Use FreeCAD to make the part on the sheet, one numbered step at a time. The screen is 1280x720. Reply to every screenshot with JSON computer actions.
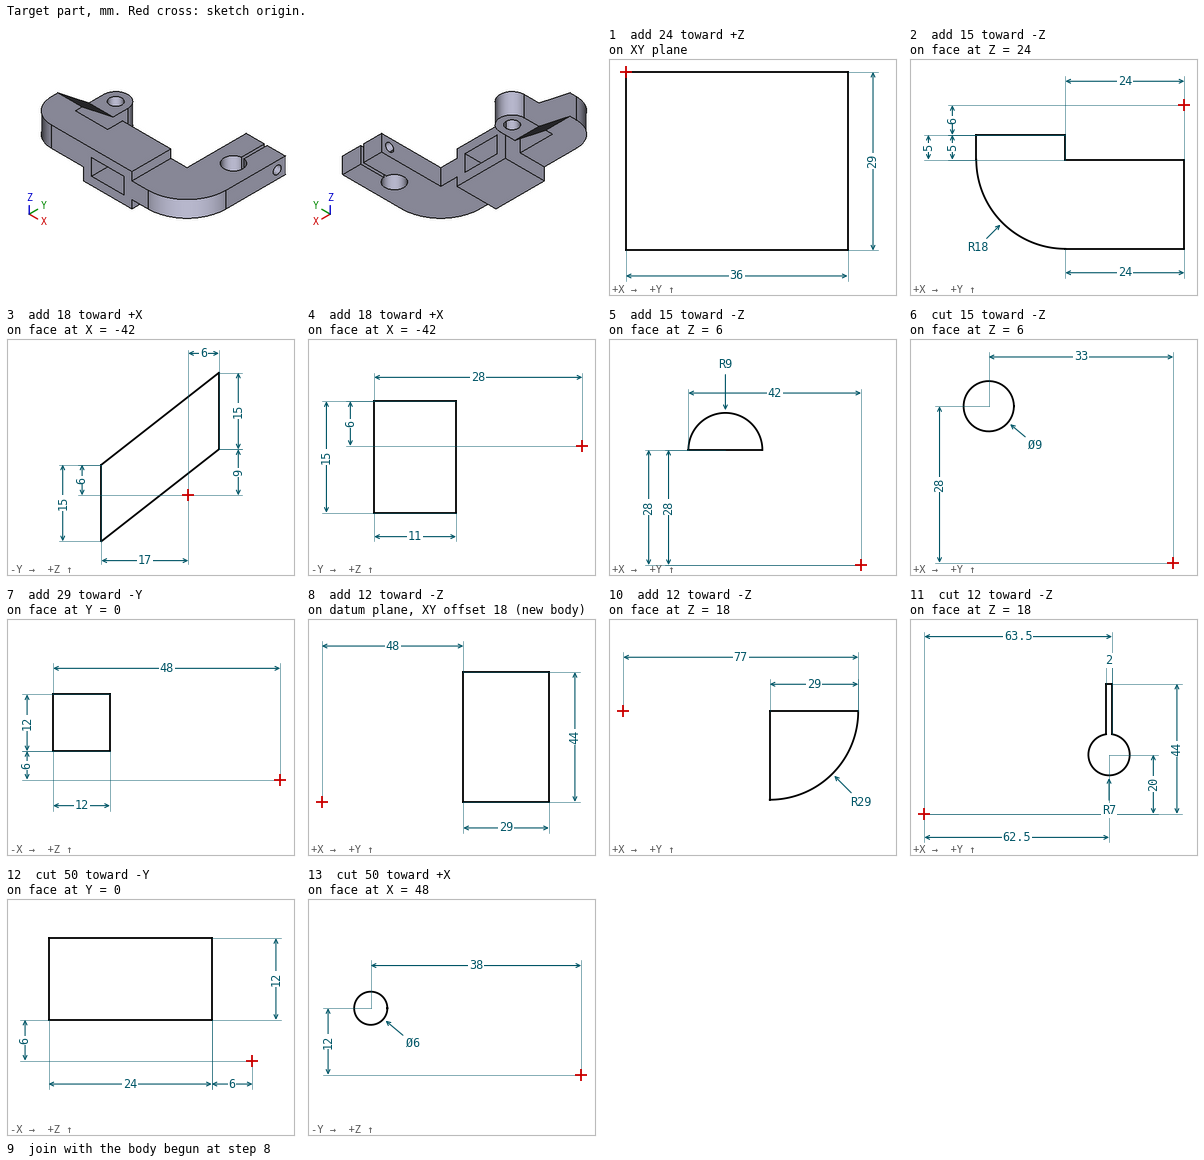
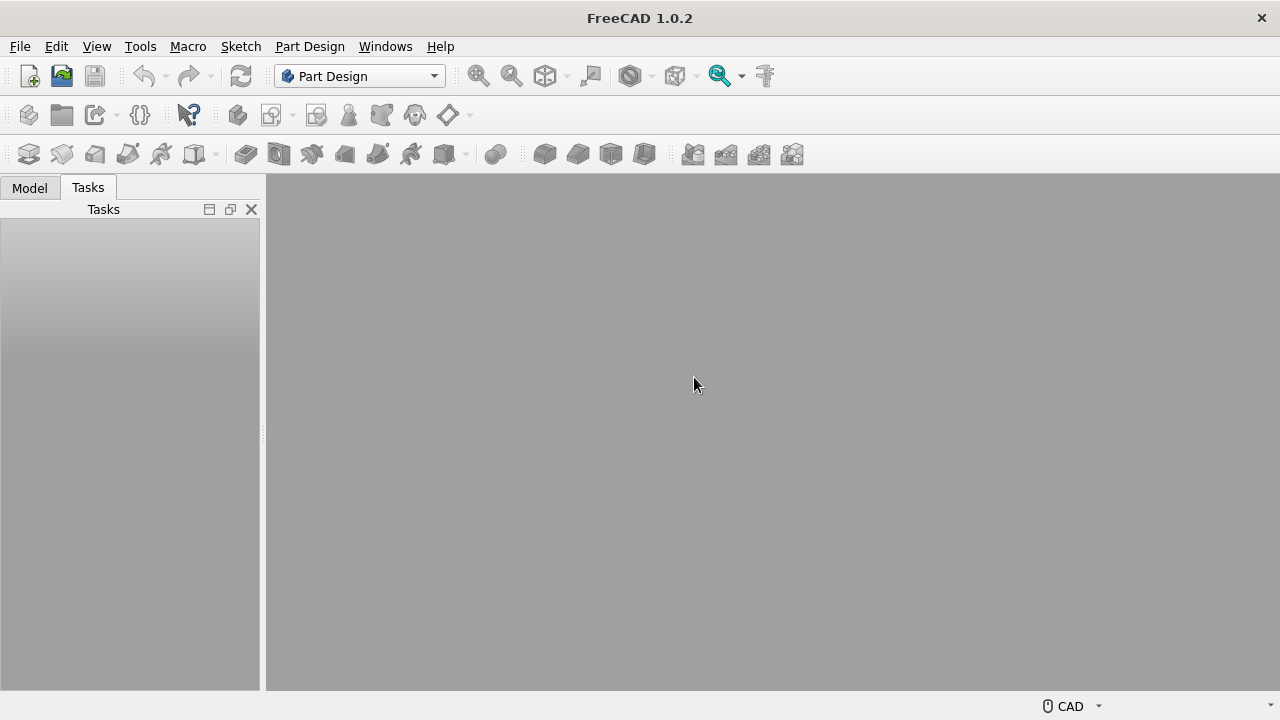
{"action": "key", "text": "ctrl+n"}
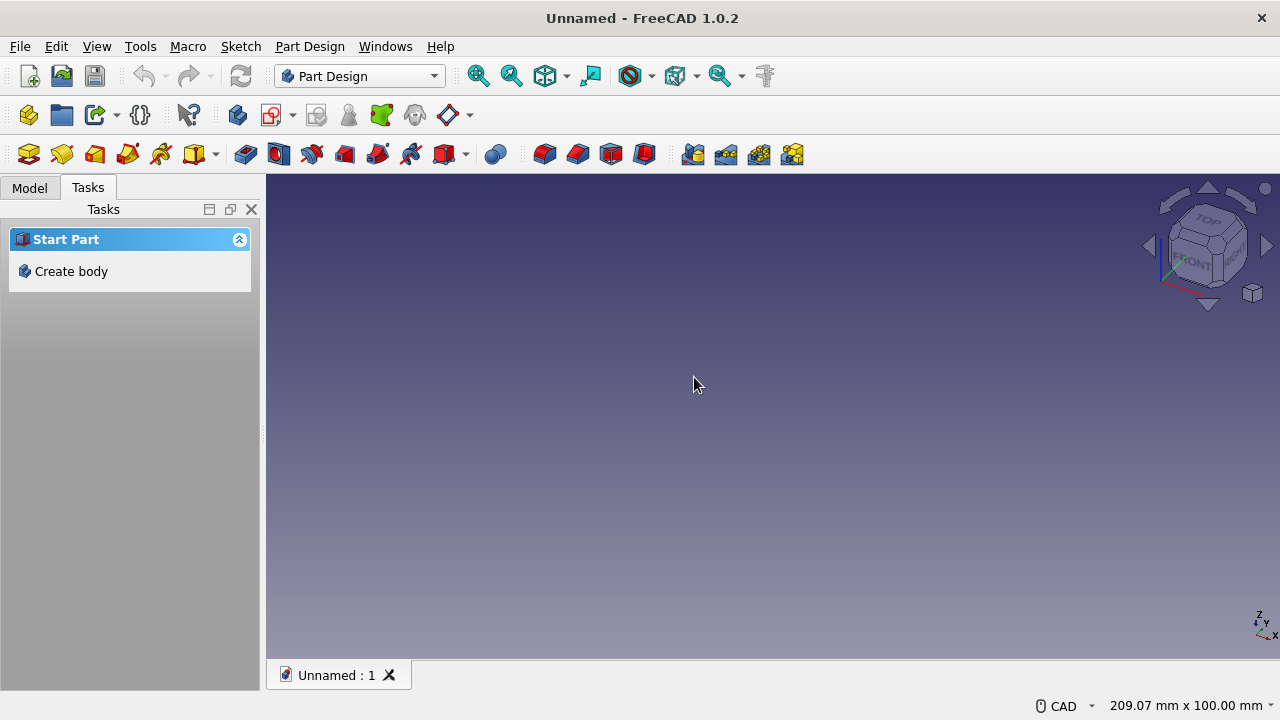
{"action": "left_click", "coordinate": [270, 116]}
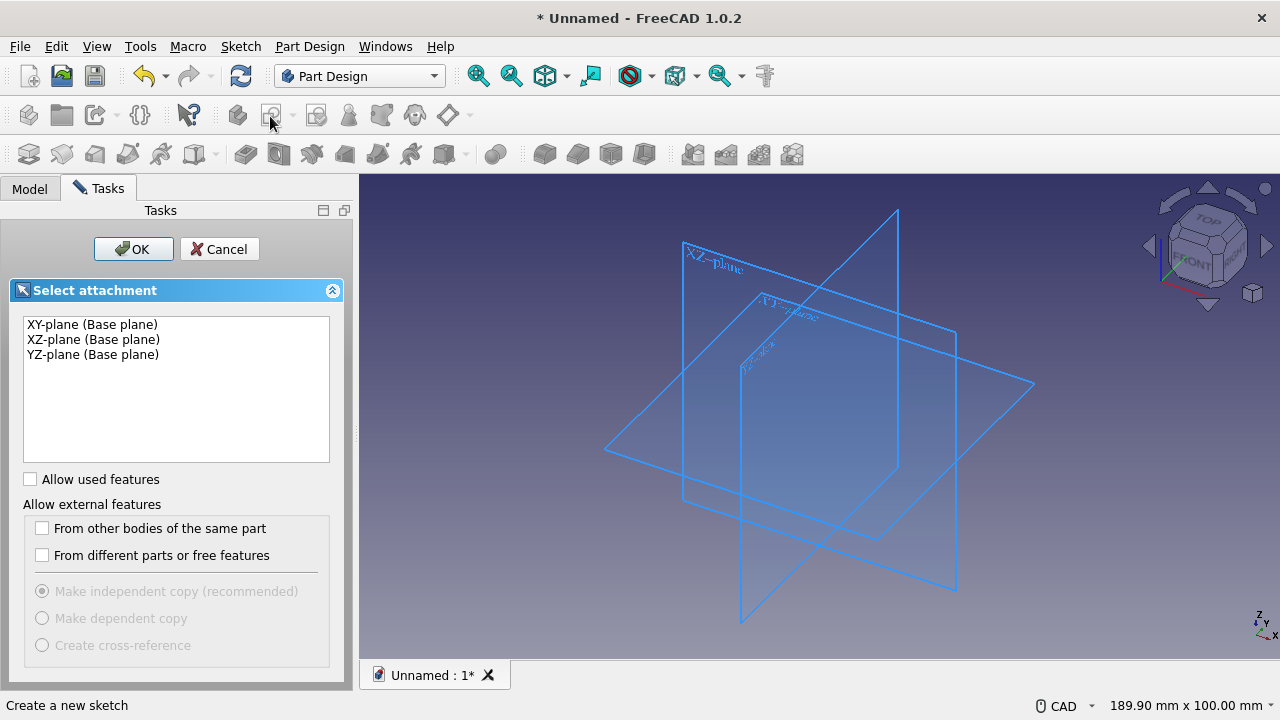
{"action": "left_click", "coordinate": [84, 324]}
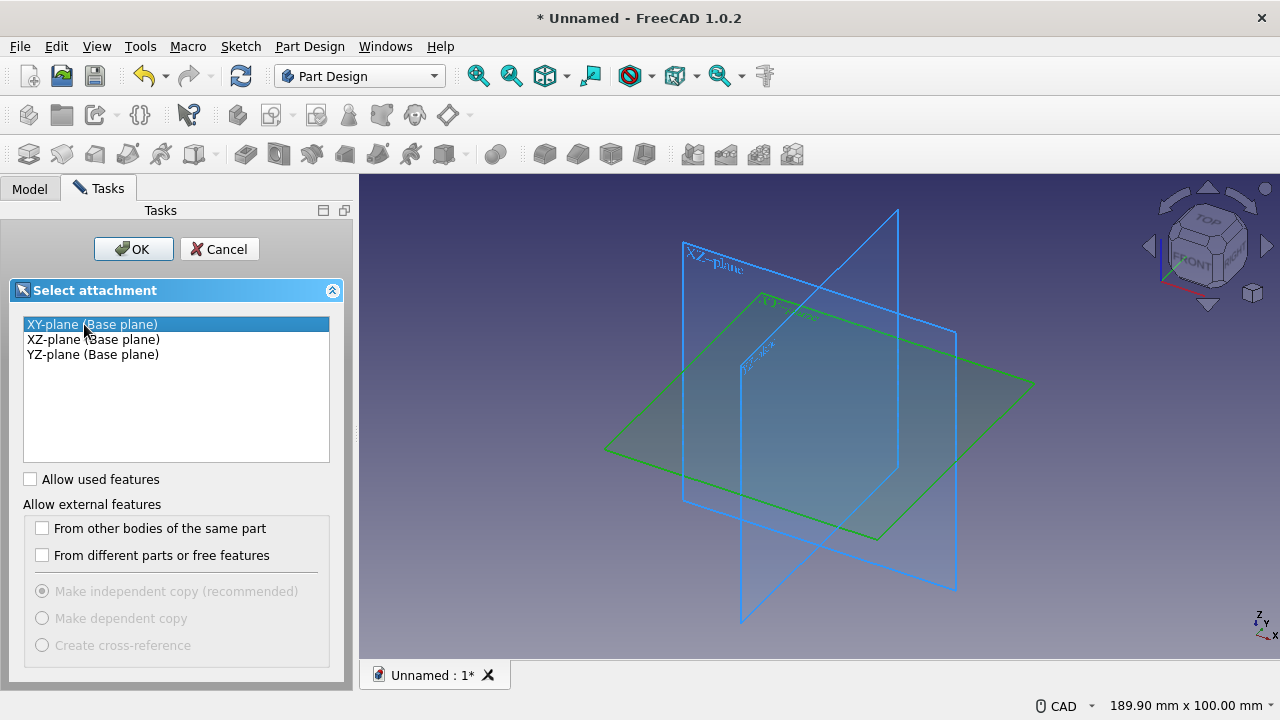
{"action": "left_click", "coordinate": [134, 249]}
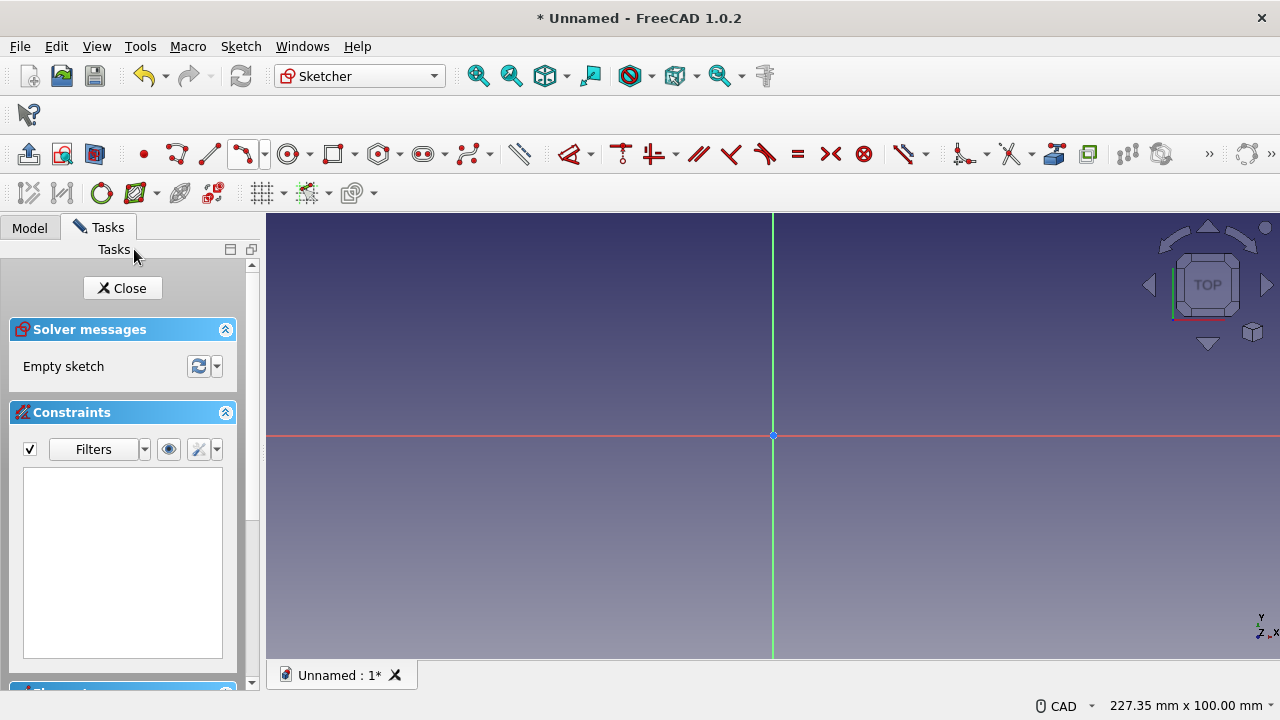
{"action": "scroll", "coordinate": [975, 553], "scroll_direction": "up", "scroll_amount": 4}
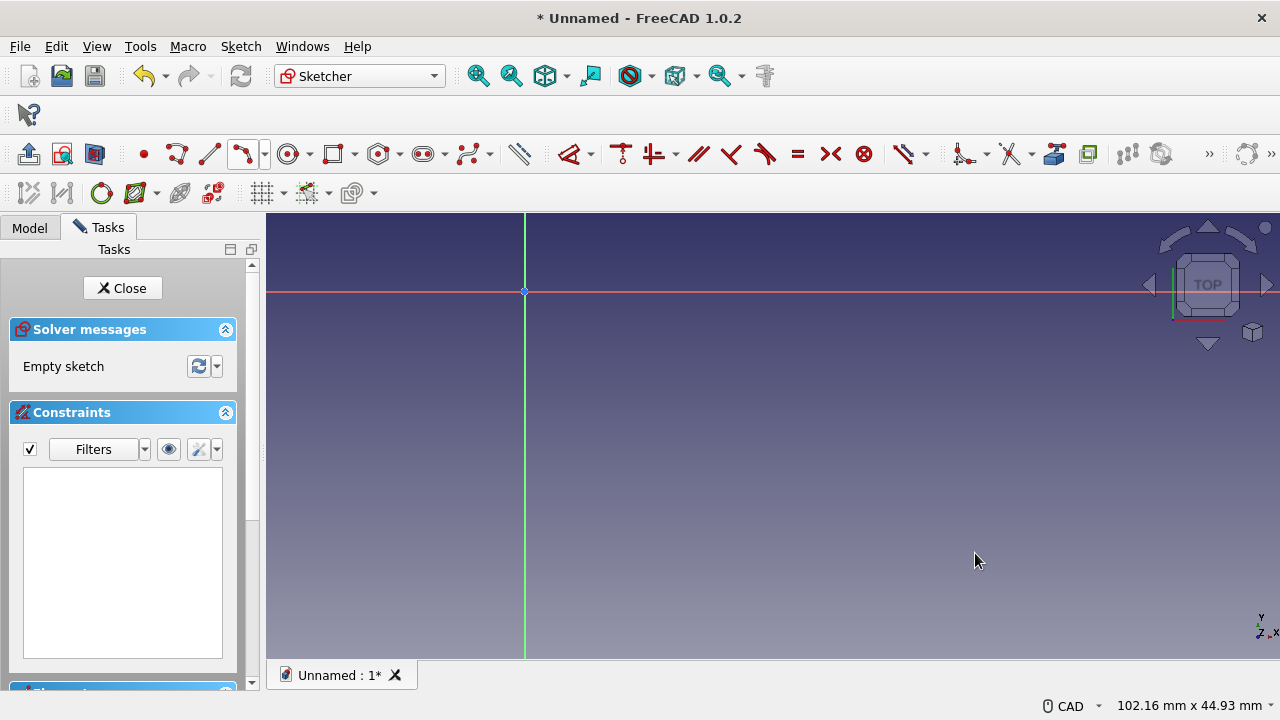
{"action": "left_click", "coordinate": [332, 154]}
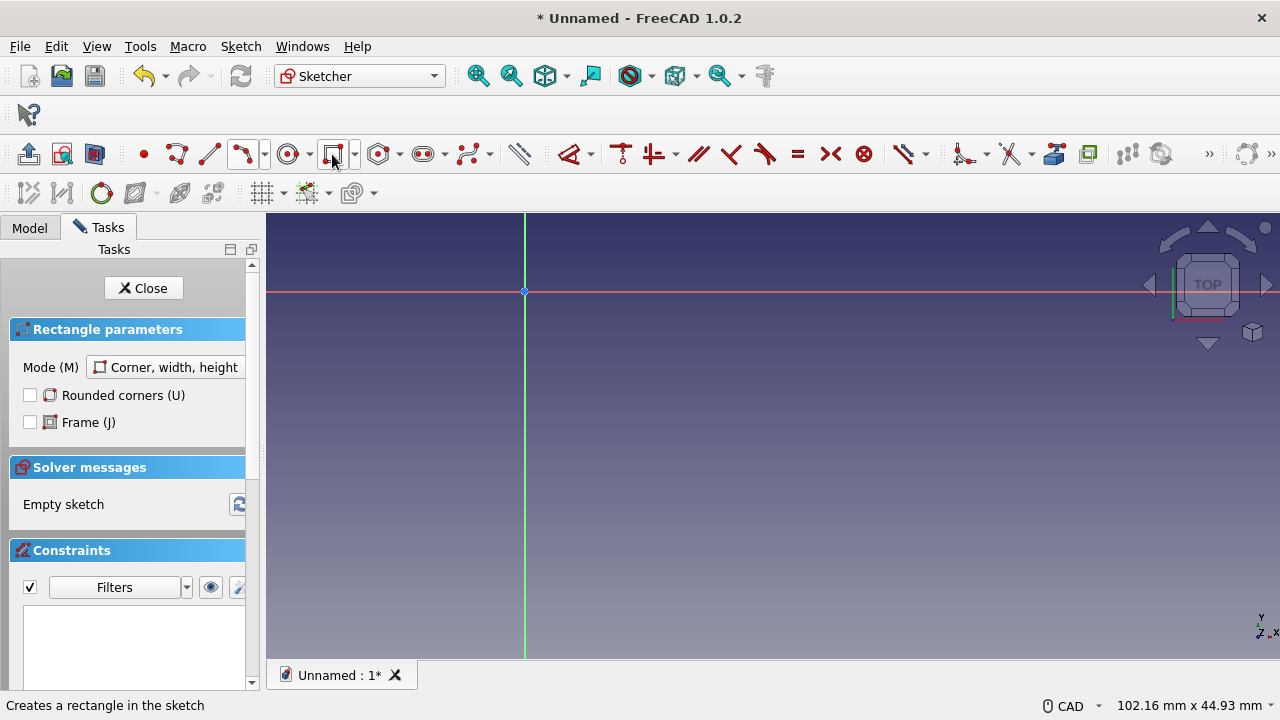
{"action": "left_click", "coordinate": [525, 292]}
{"action": "mouse_move", "coordinate": [882, 580]}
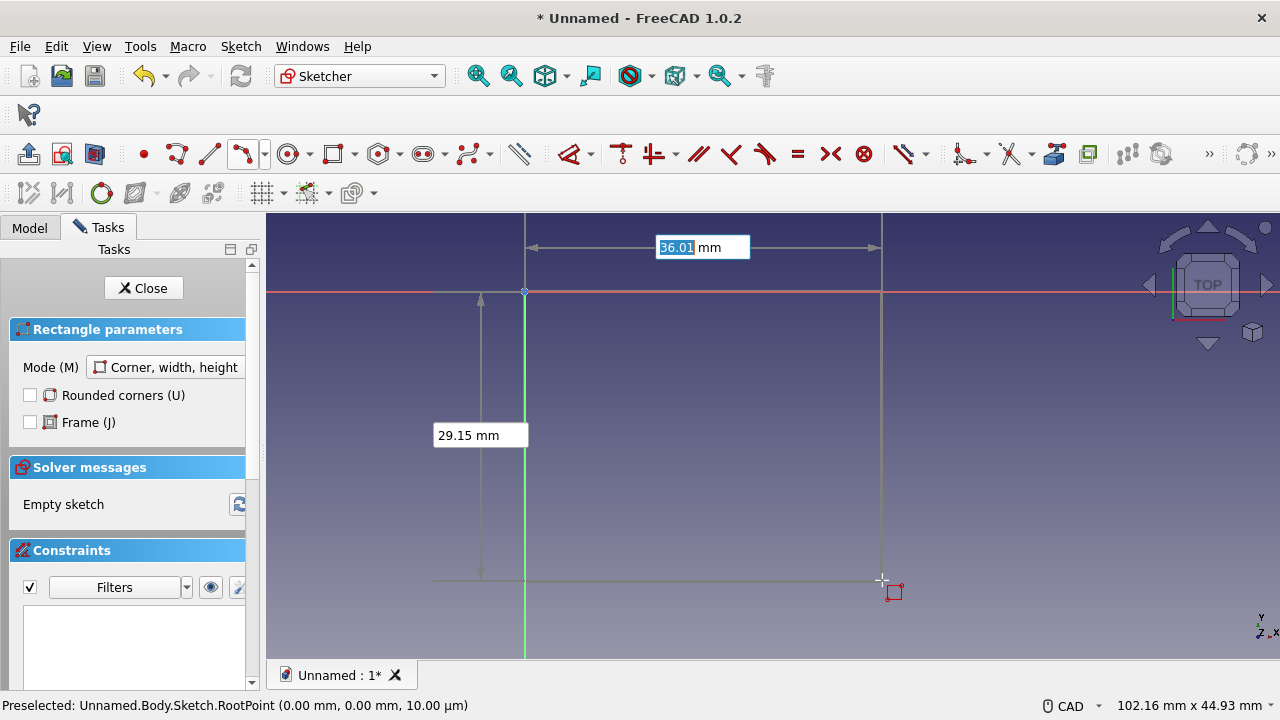
{"action": "type", "text": "36"}
{"action": "key", "text": "Tab"}
{"action": "type", "text": "29"}
{"action": "key", "text": "Return"}
{"action": "key", "text": "Escape"}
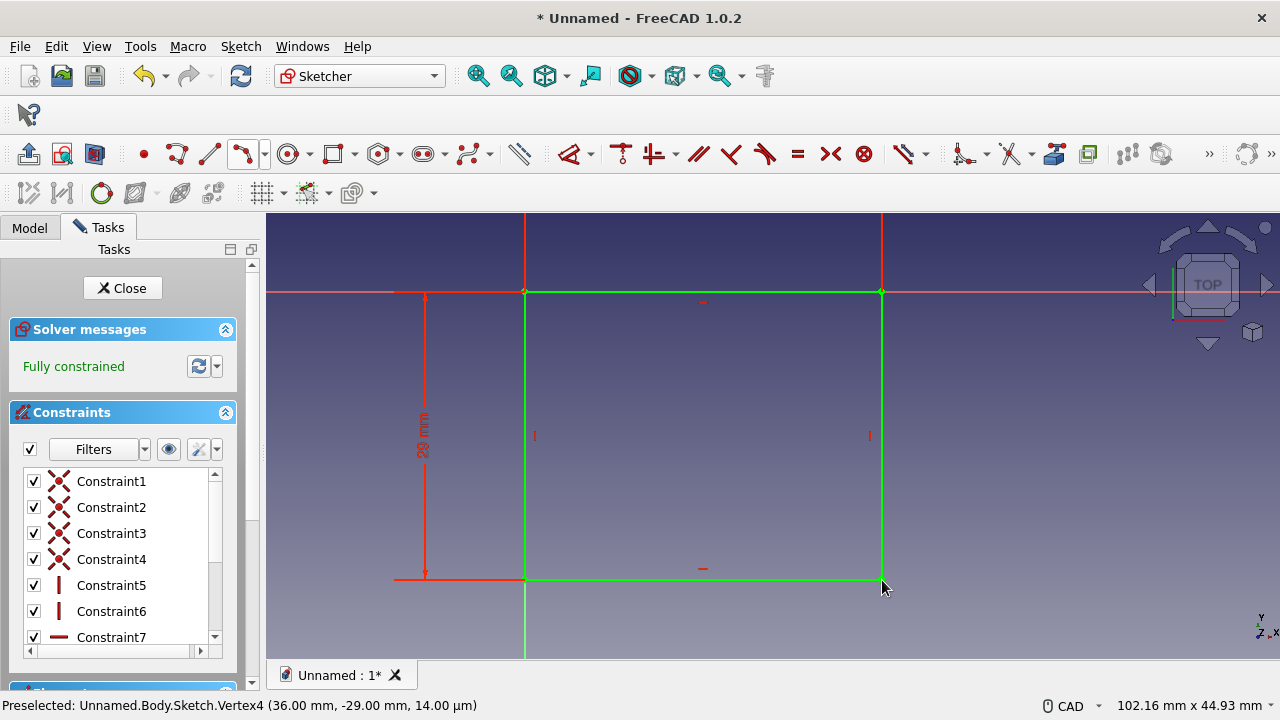
{"action": "left_click", "coordinate": [123, 288]}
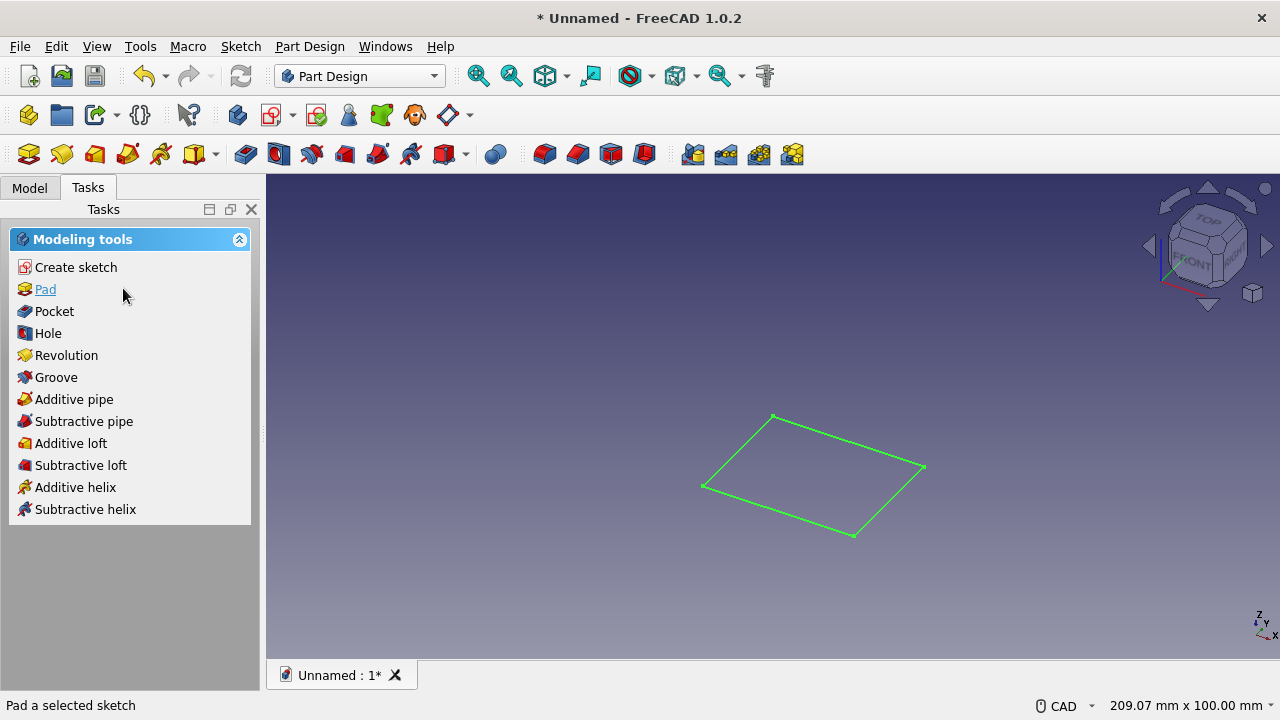
{"action": "left_click", "coordinate": [29, 154]}